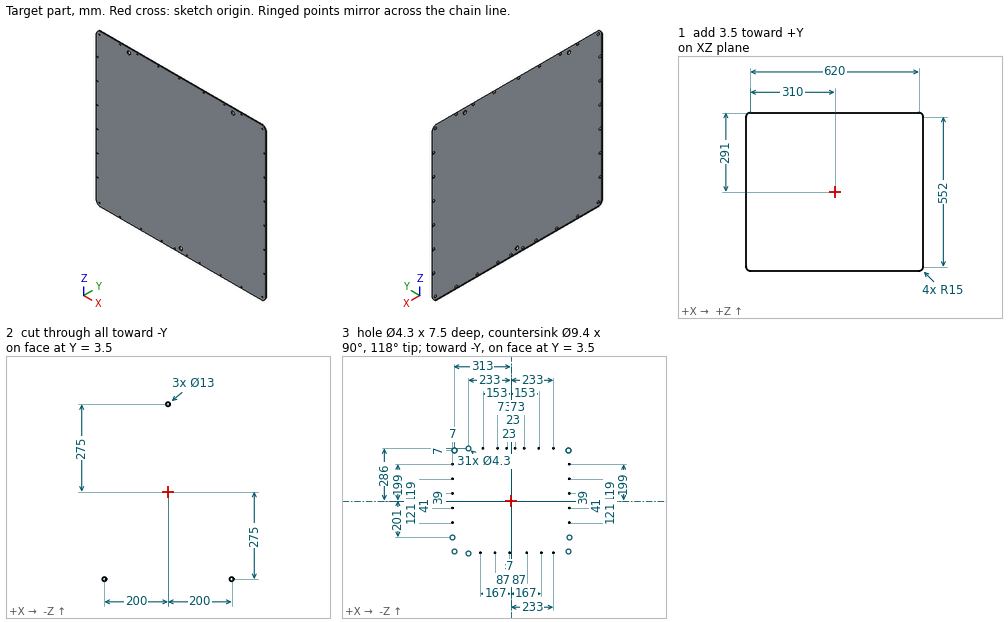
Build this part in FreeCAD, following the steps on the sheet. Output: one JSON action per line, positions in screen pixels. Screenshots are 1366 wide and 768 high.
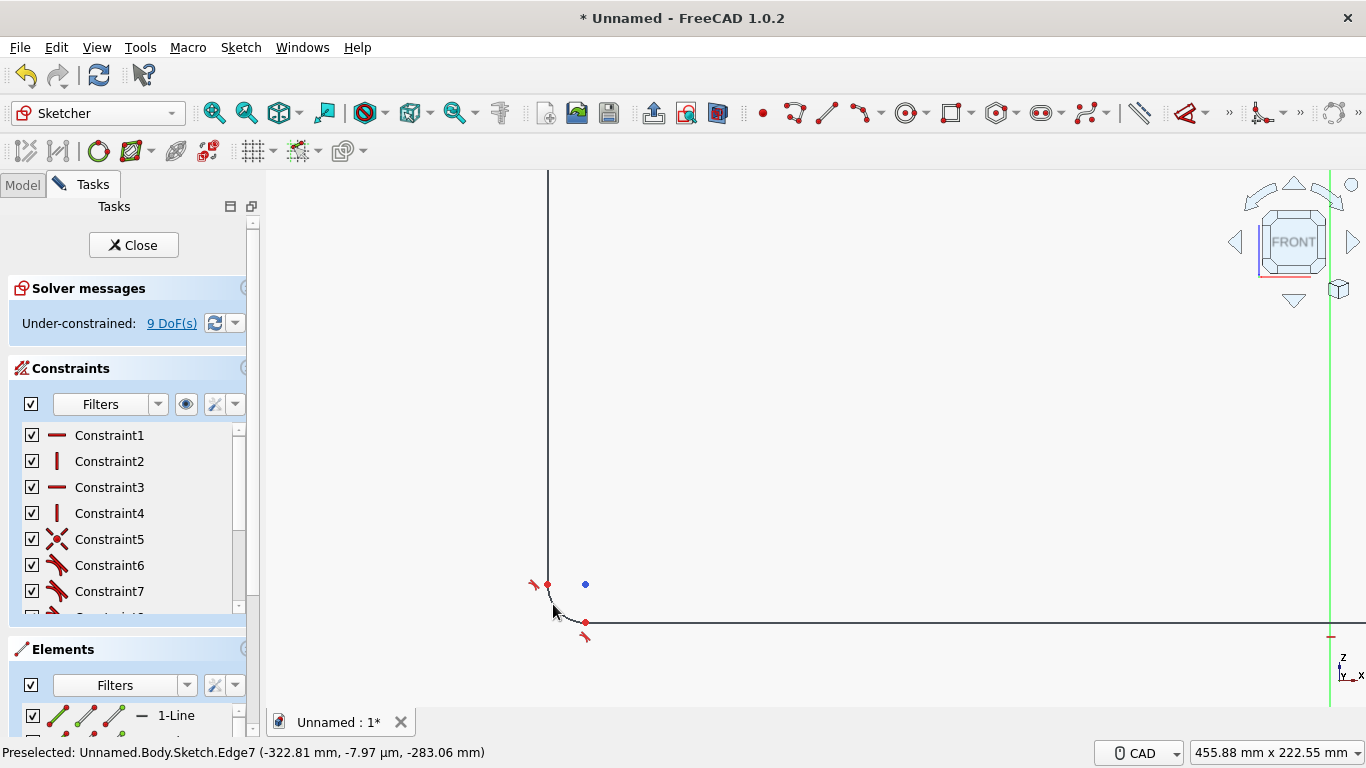
{"action": "scroll", "coordinate": [557, 609], "scroll_direction": "down", "scroll_amount": 7}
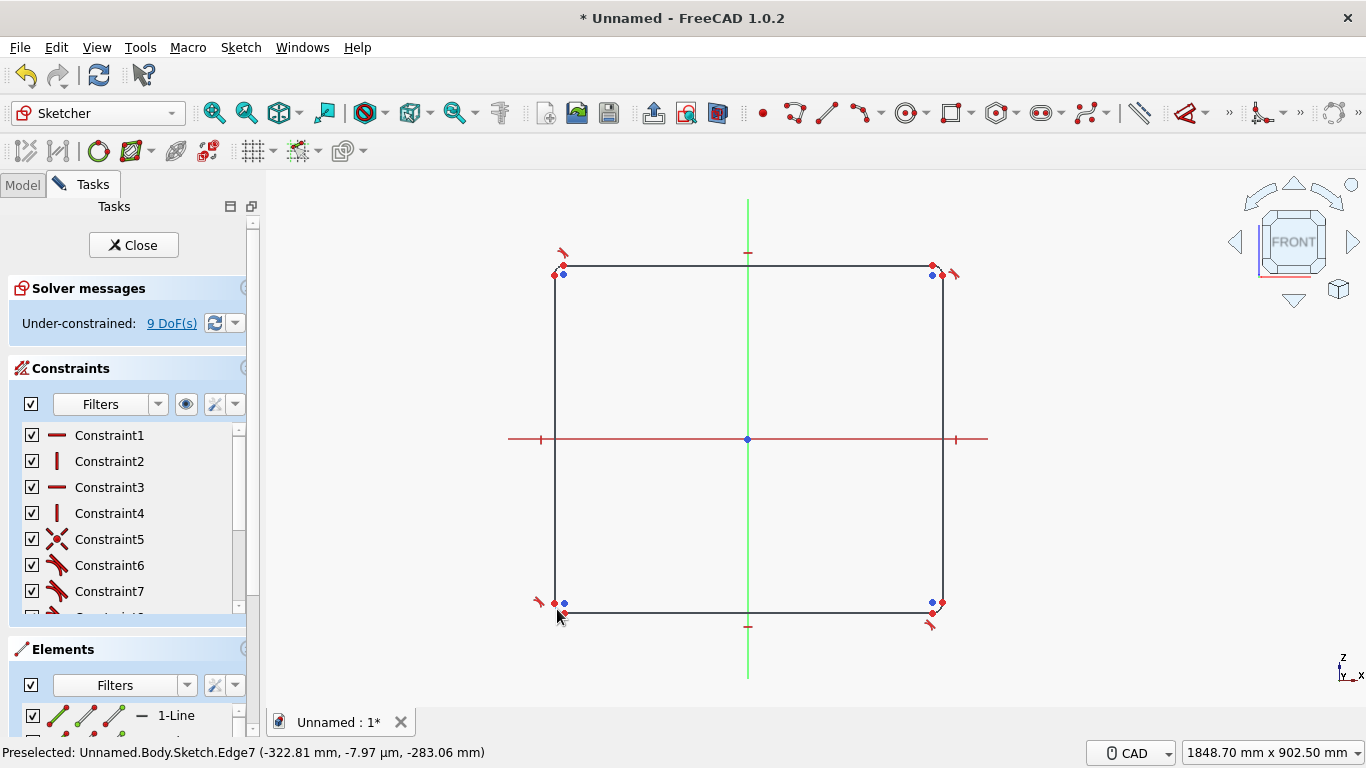
{"action": "left_click", "coordinate": [555, 538]}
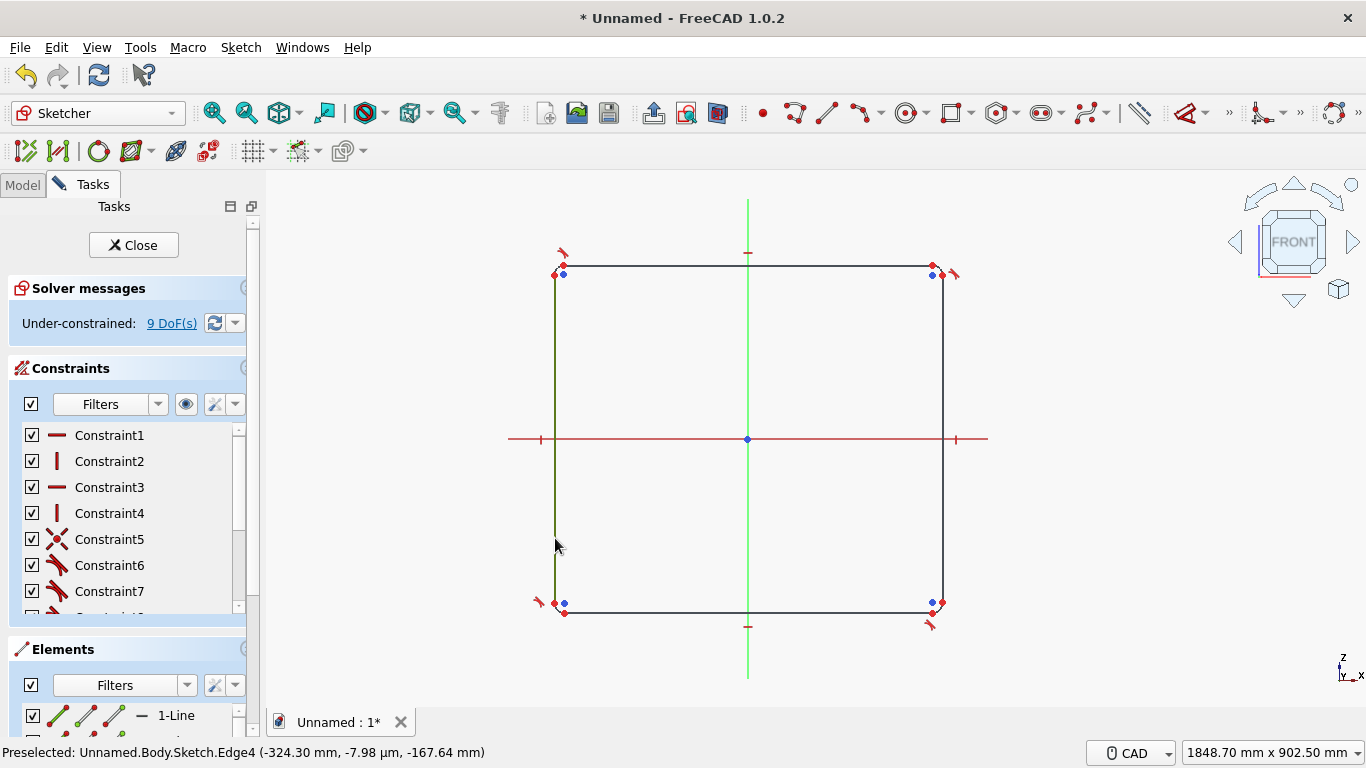
{"action": "scroll", "coordinate": [557, 269], "scroll_direction": "up", "scroll_amount": 4}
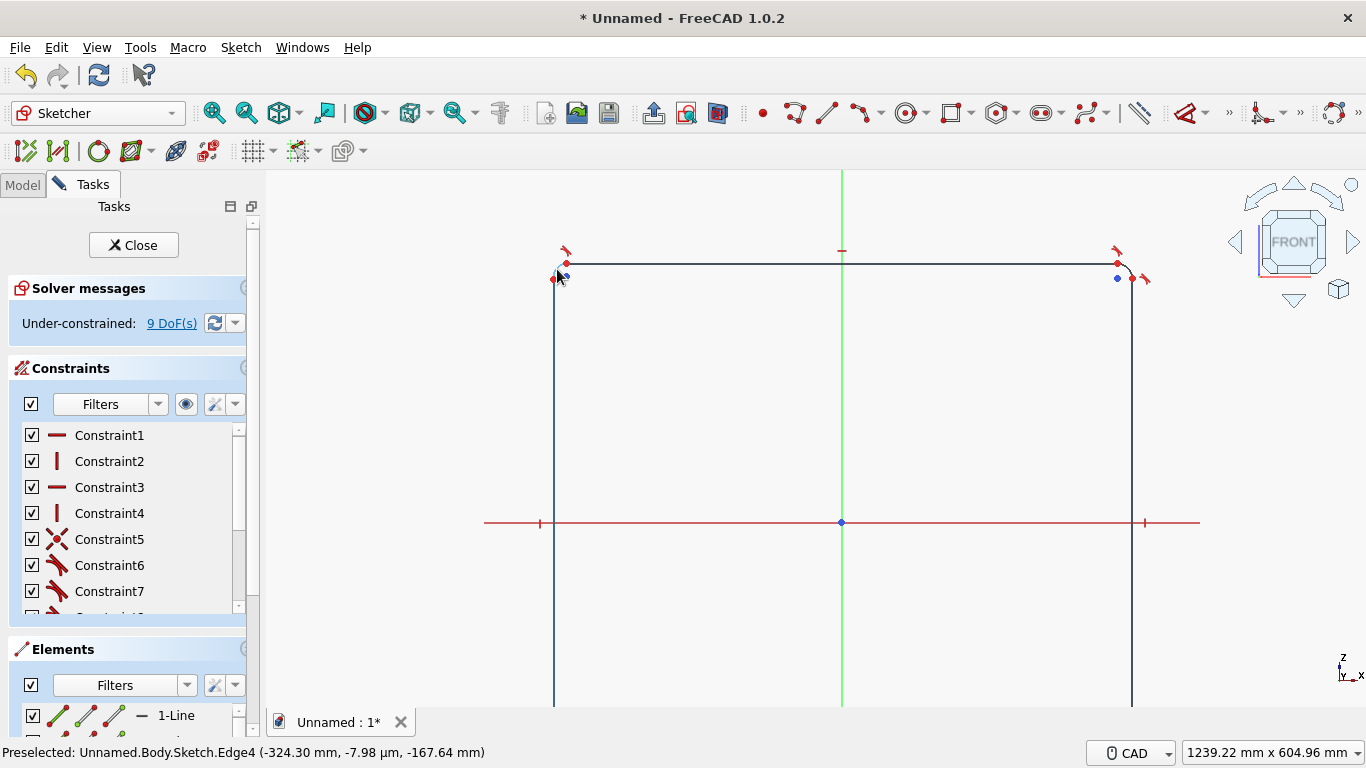
{"action": "left_click", "coordinate": [557, 268]}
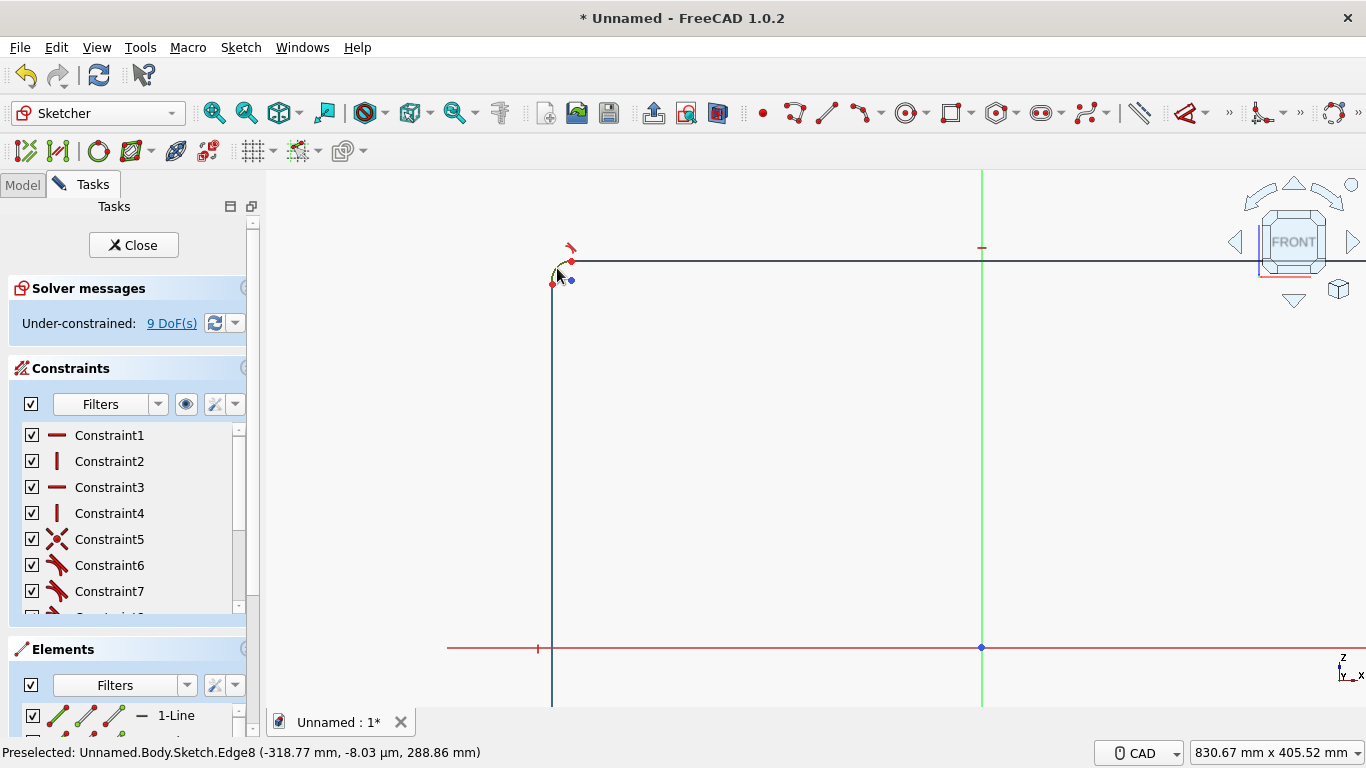
{"action": "key", "text": "t"}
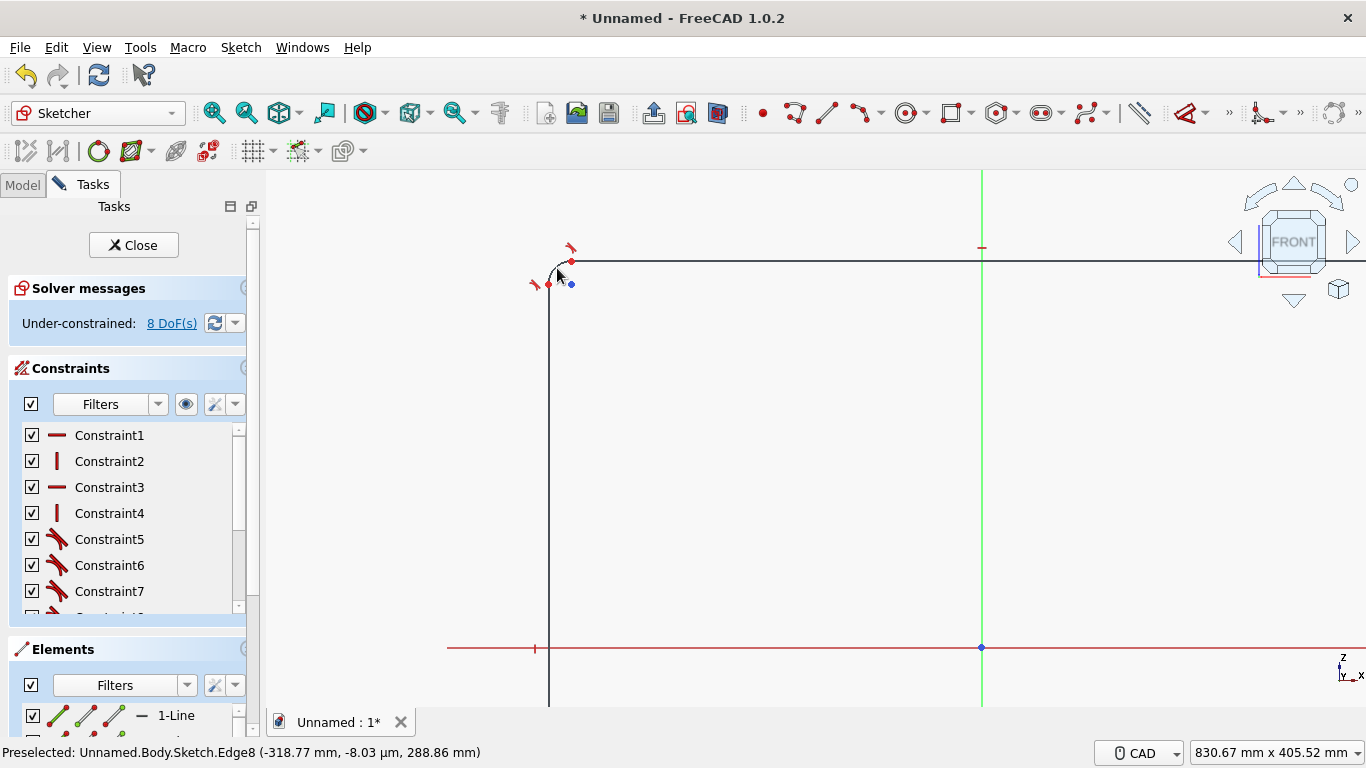
{"action": "scroll", "coordinate": [556, 268], "scroll_direction": "down", "scroll_amount": 4}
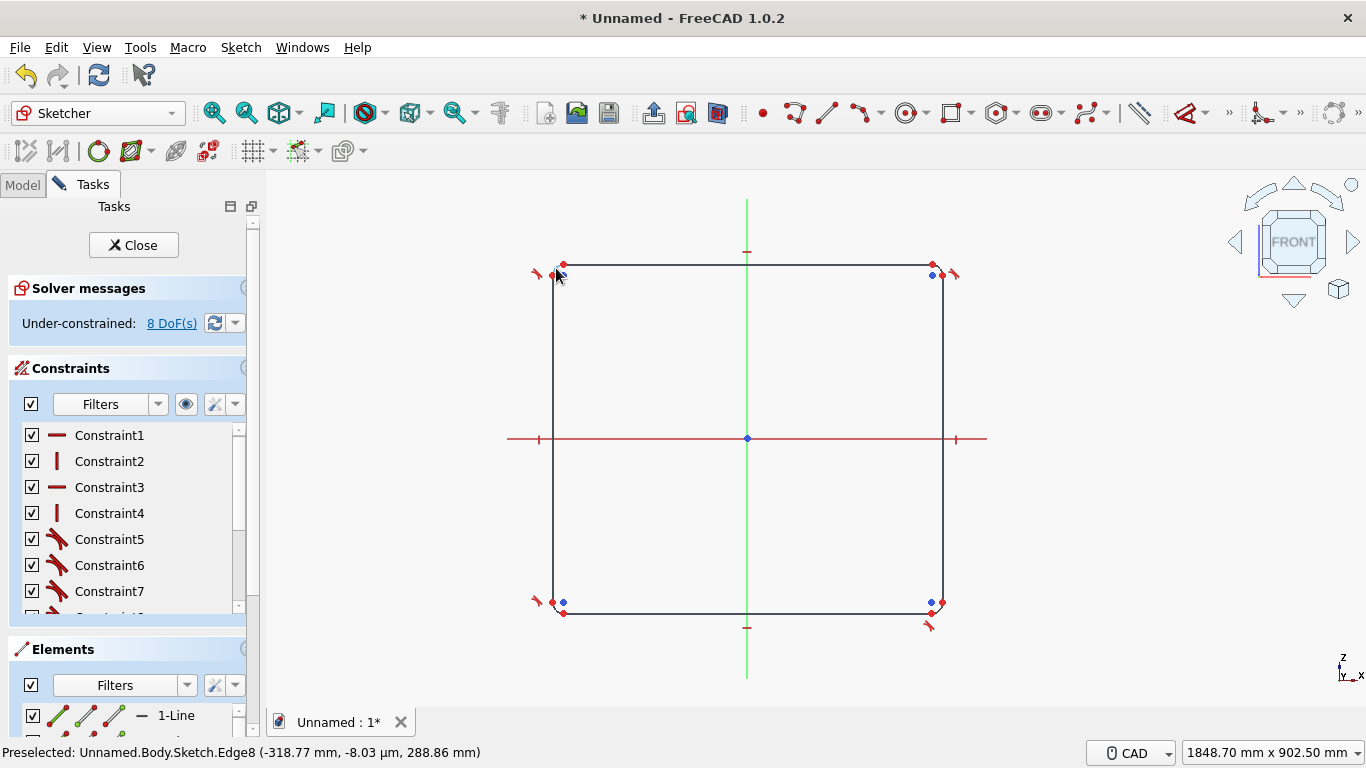
{"action": "scroll", "coordinate": [941, 271], "scroll_direction": "up", "scroll_amount": 6}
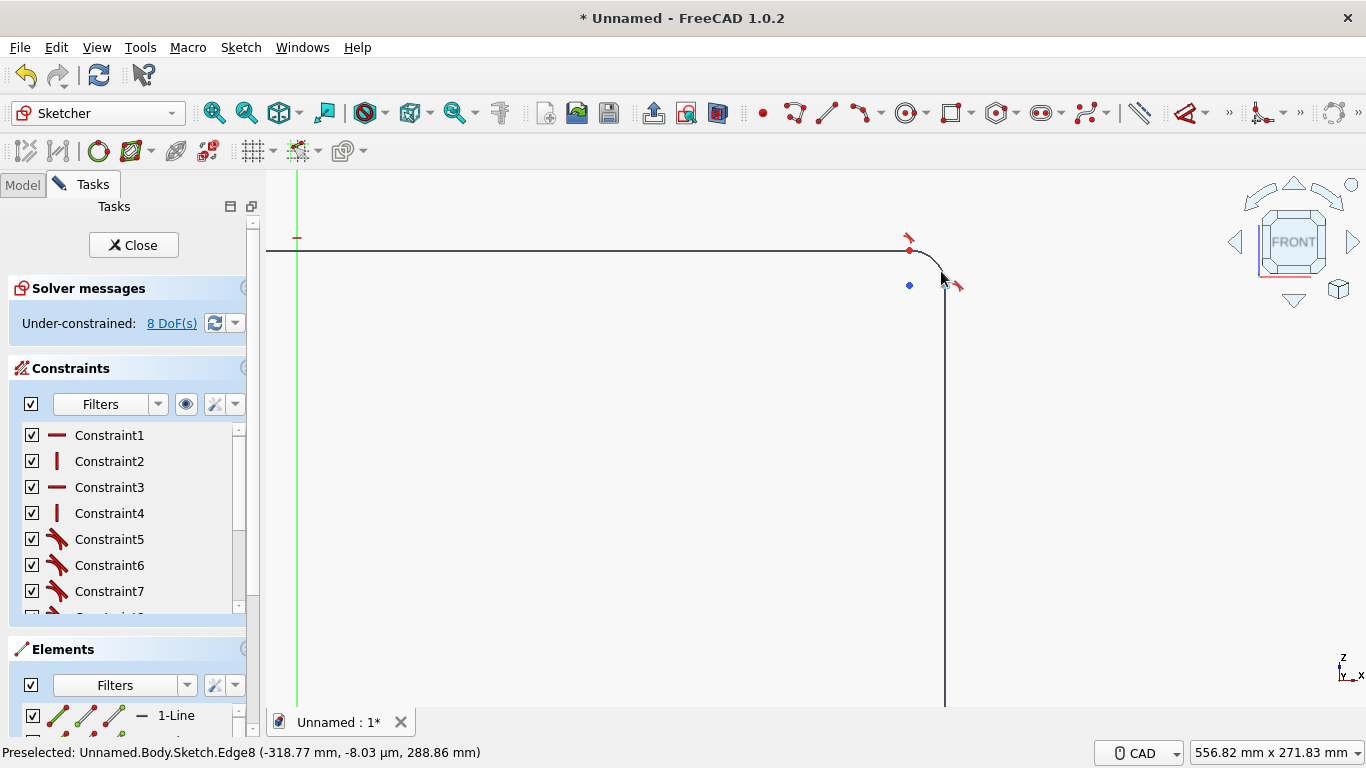
{"action": "left_click", "coordinate": [941, 270]}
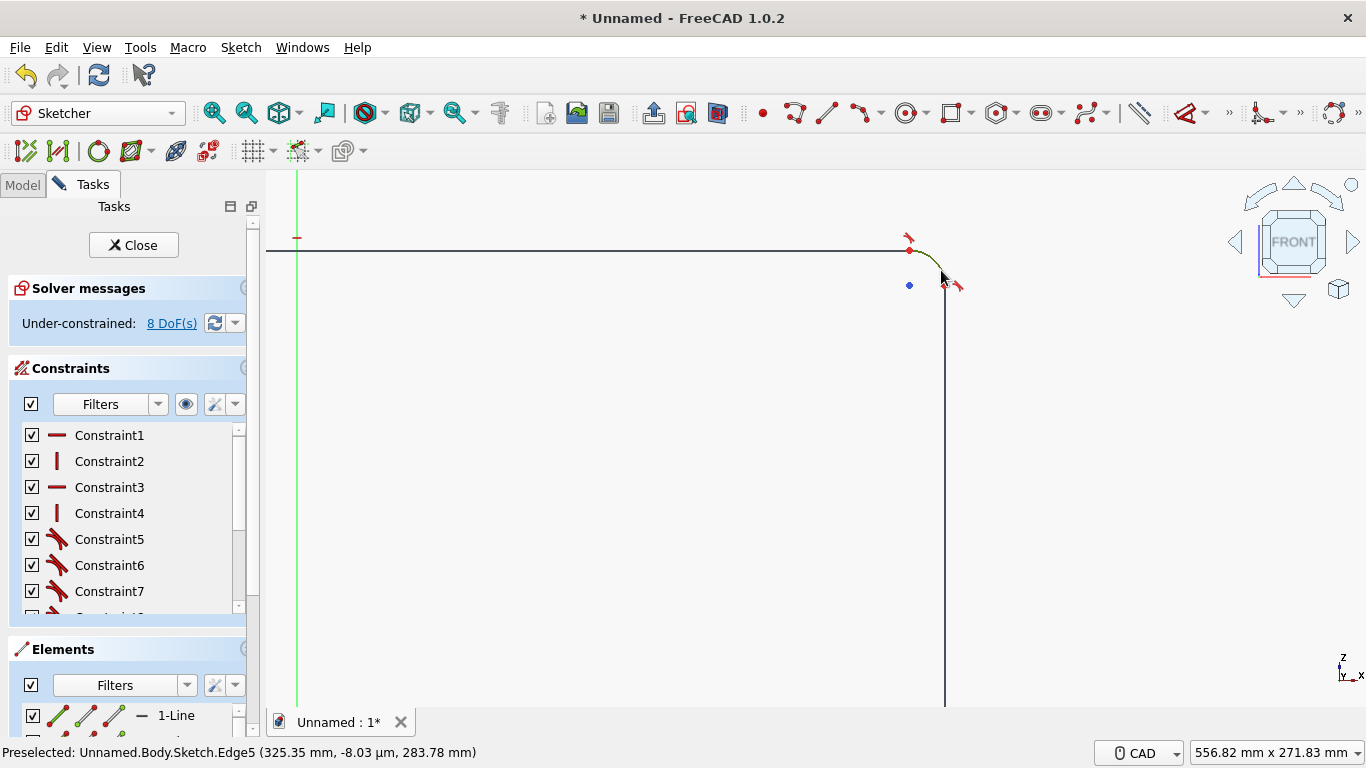
{"action": "scroll", "coordinate": [942, 271], "scroll_direction": "down", "scroll_amount": 6}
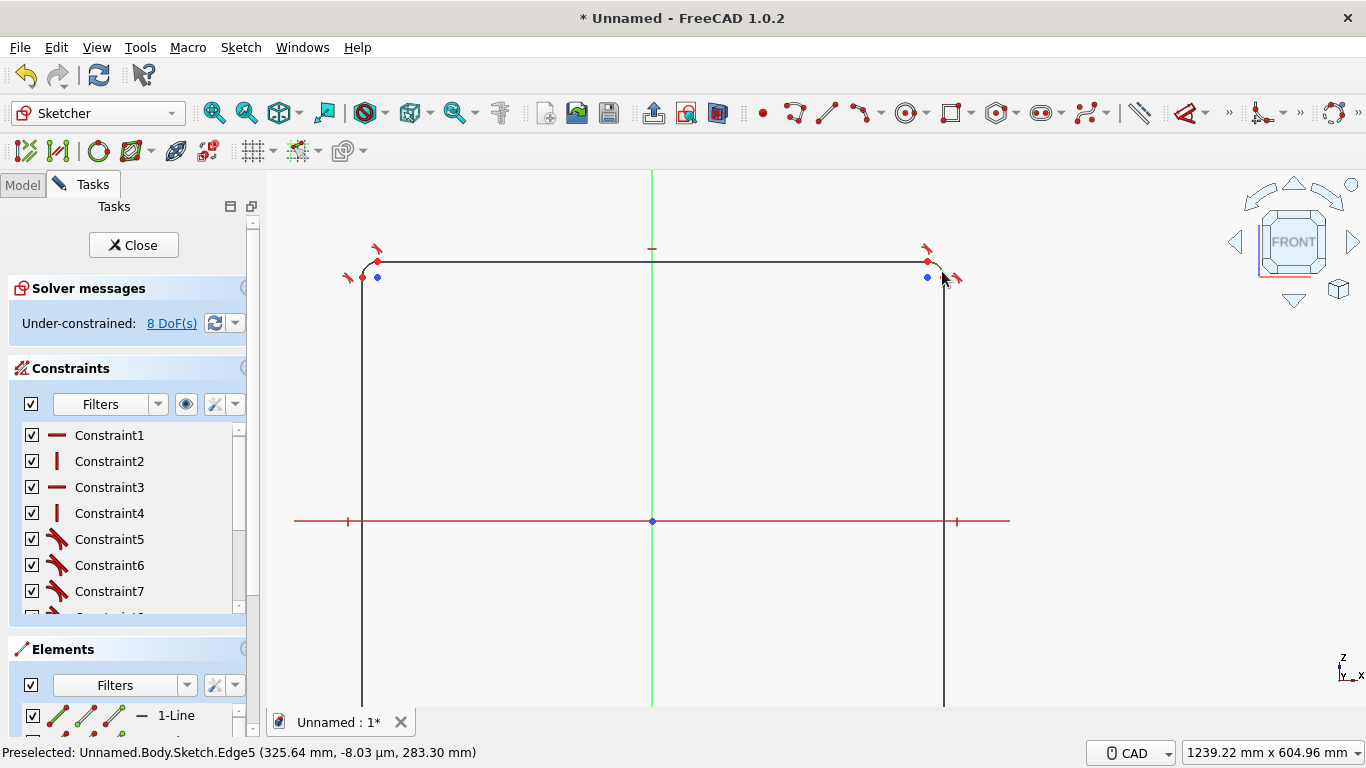
{"action": "scroll", "coordinate": [937, 612], "scroll_direction": "up", "scroll_amount": 5}